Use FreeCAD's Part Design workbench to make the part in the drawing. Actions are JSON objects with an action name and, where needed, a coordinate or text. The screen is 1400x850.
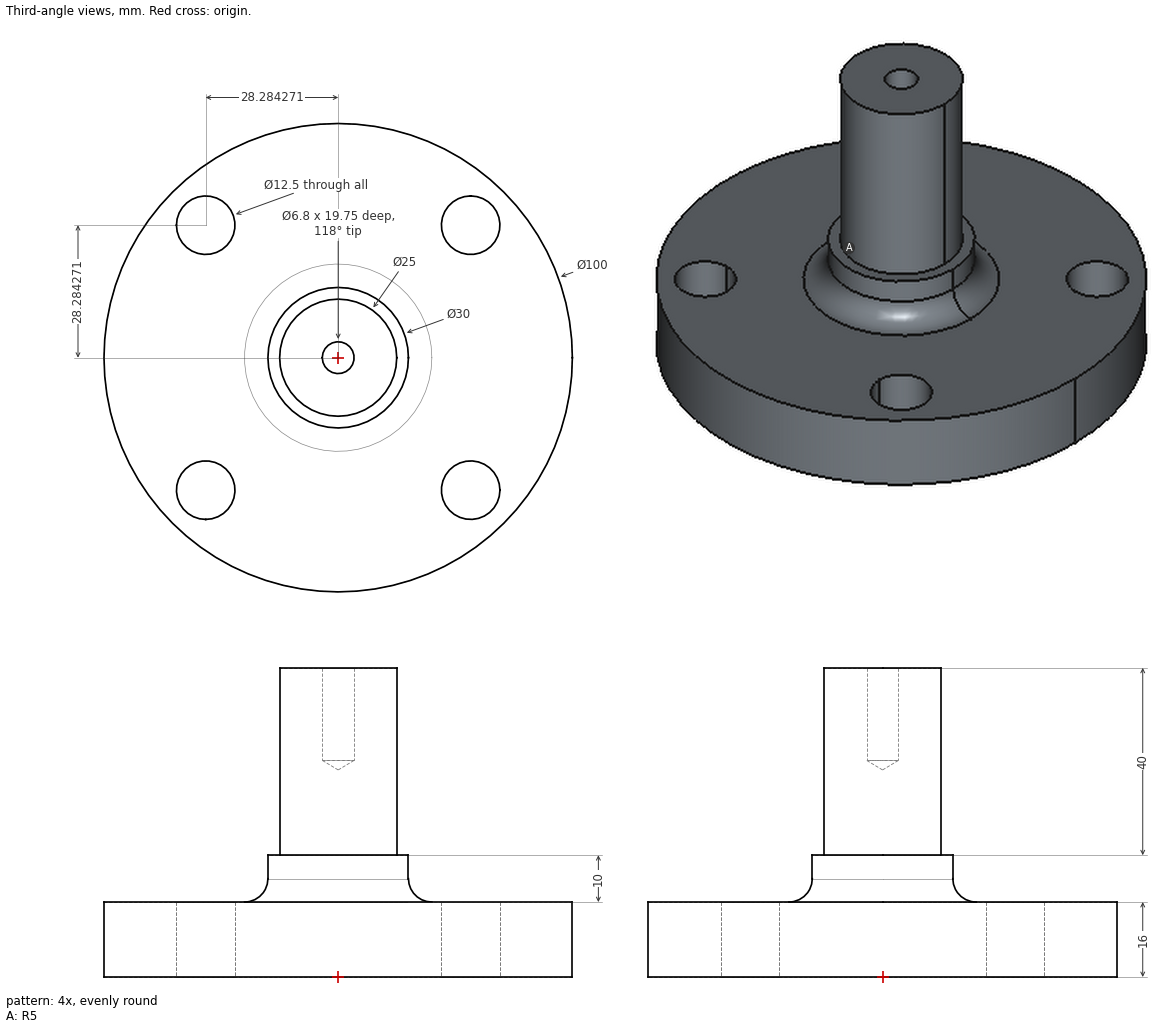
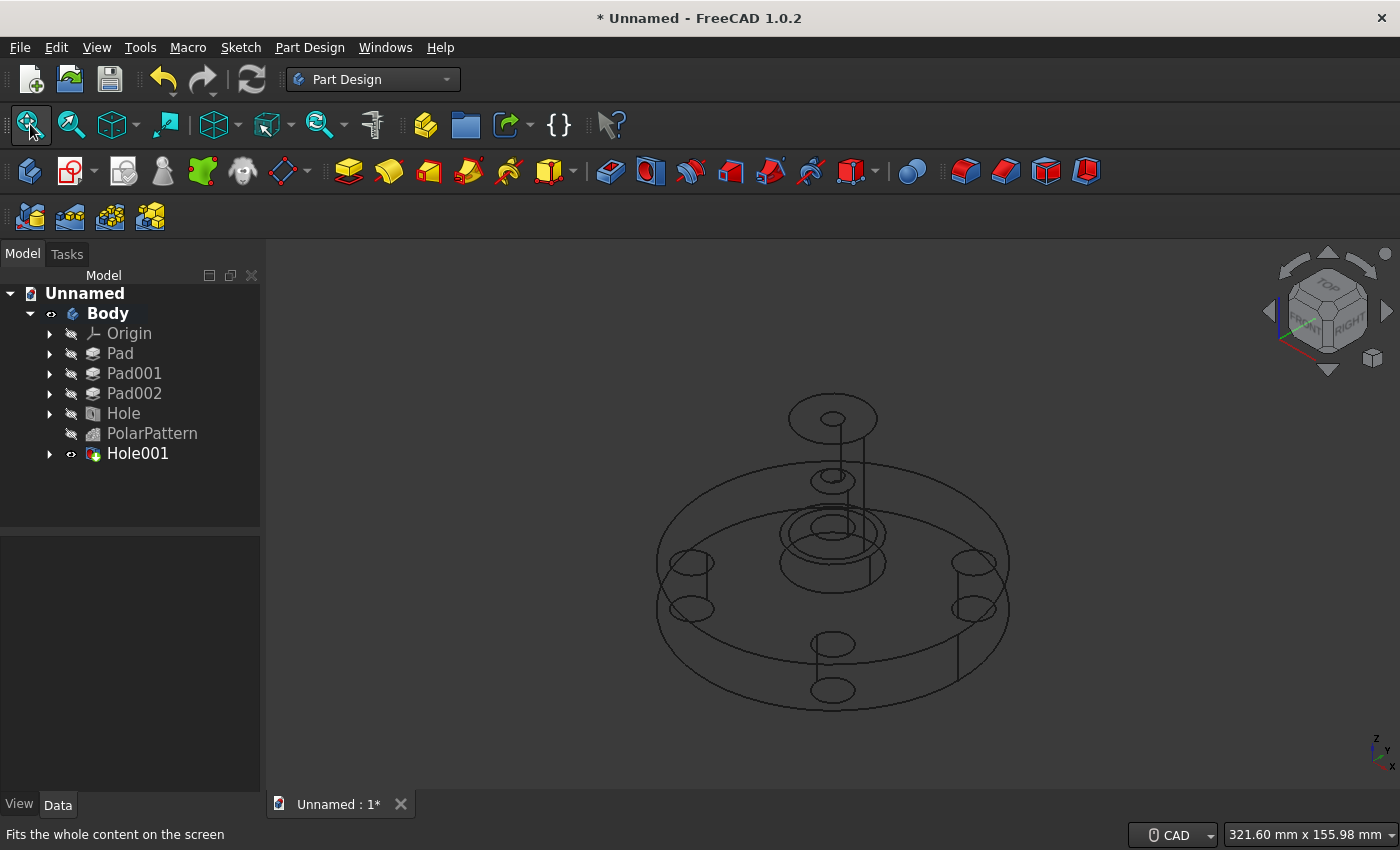
{"action": "left_click", "coordinate": [825, 532]}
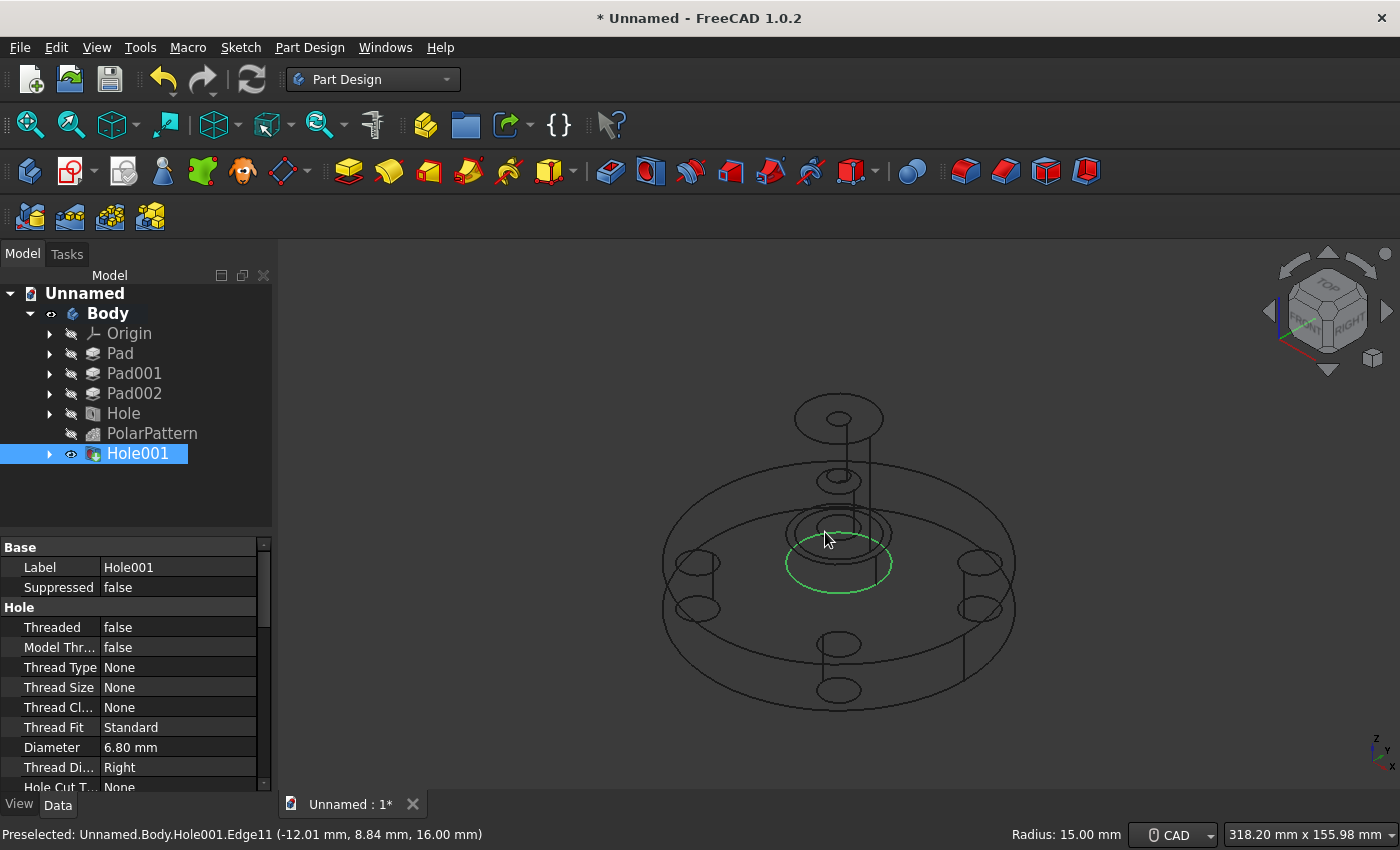
{"action": "key", "text": "v 1"}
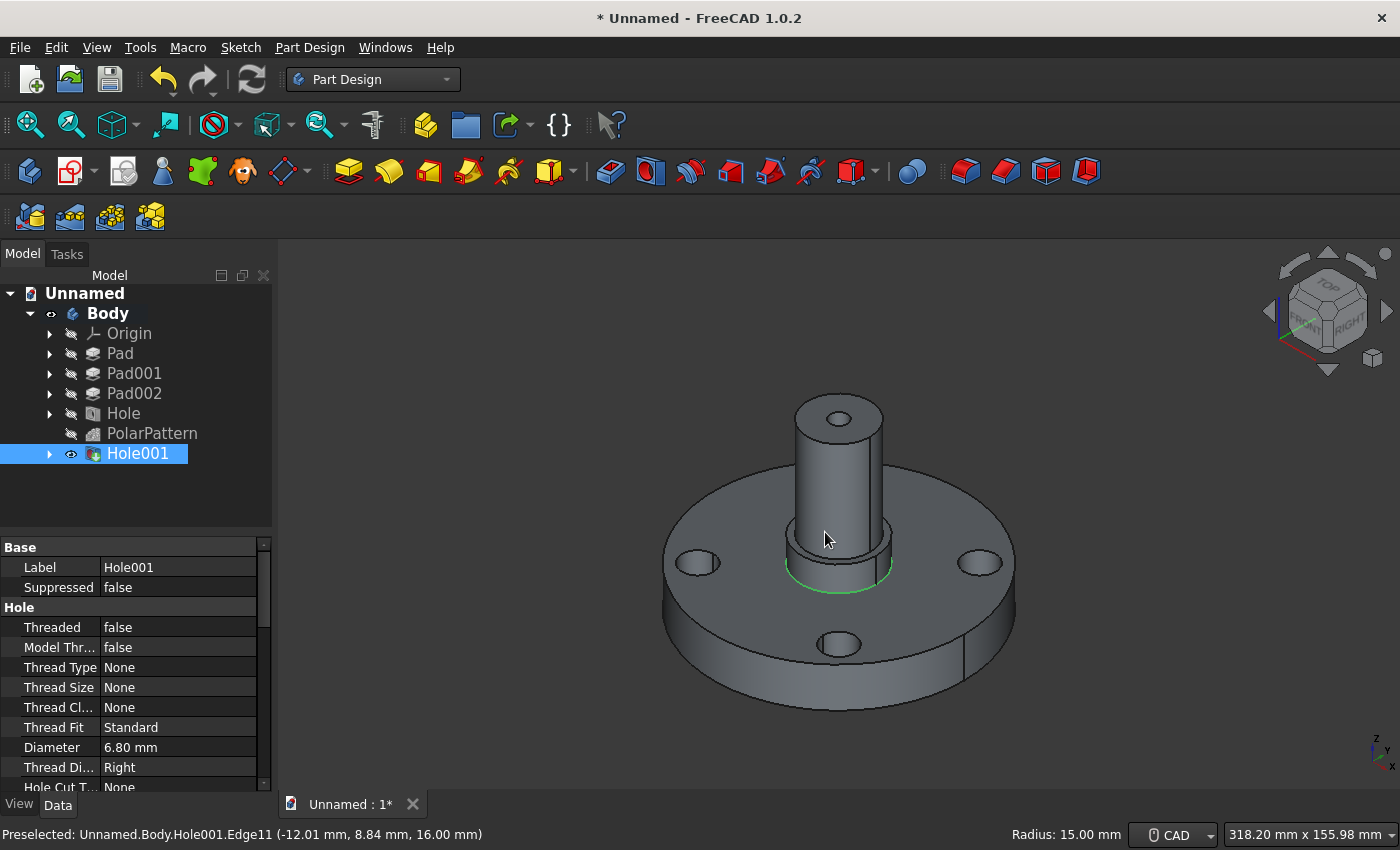
{"action": "left_click", "coordinate": [966, 172]}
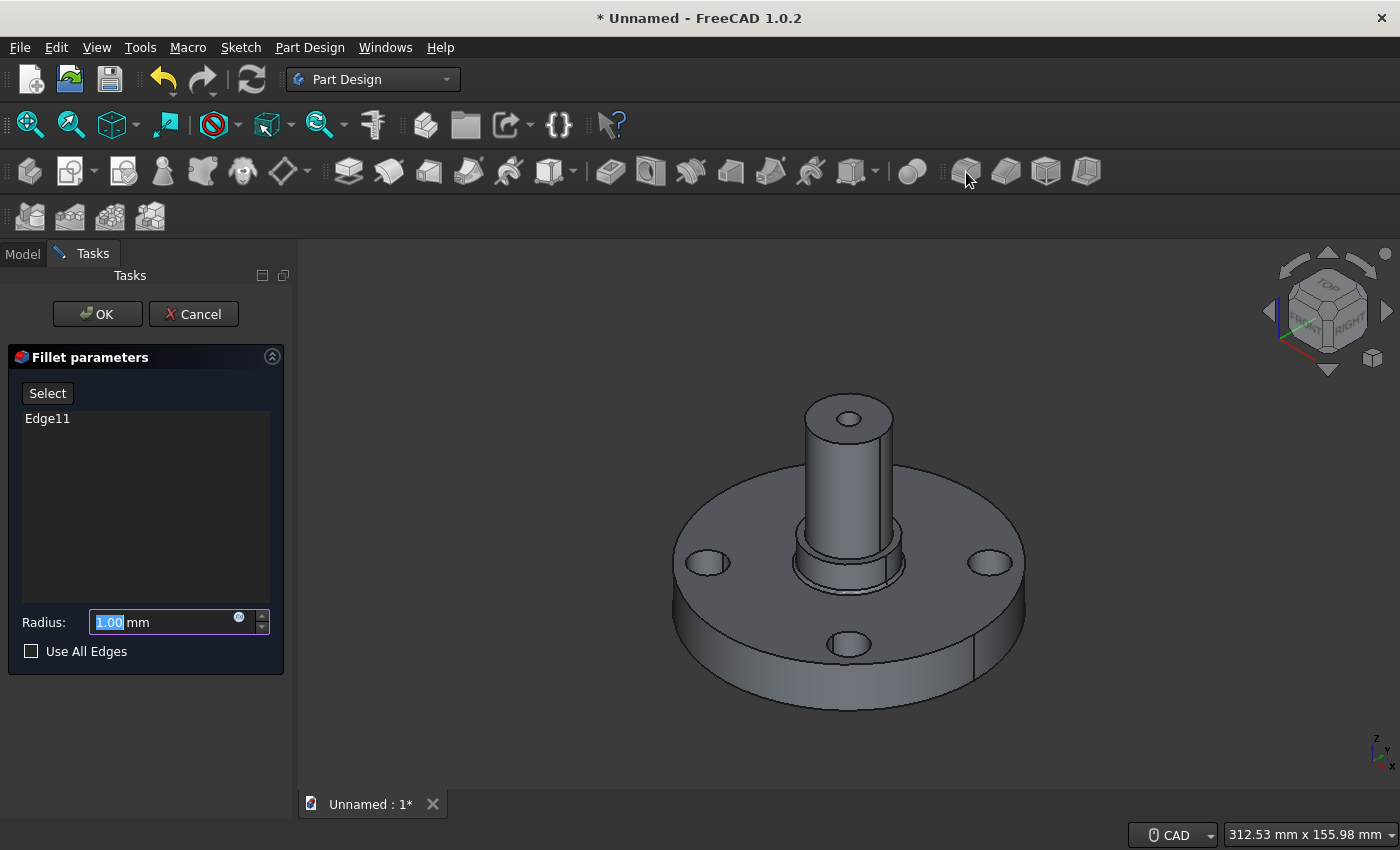
{"action": "type", "text": "5"}
{"action": "key", "text": "Tab"}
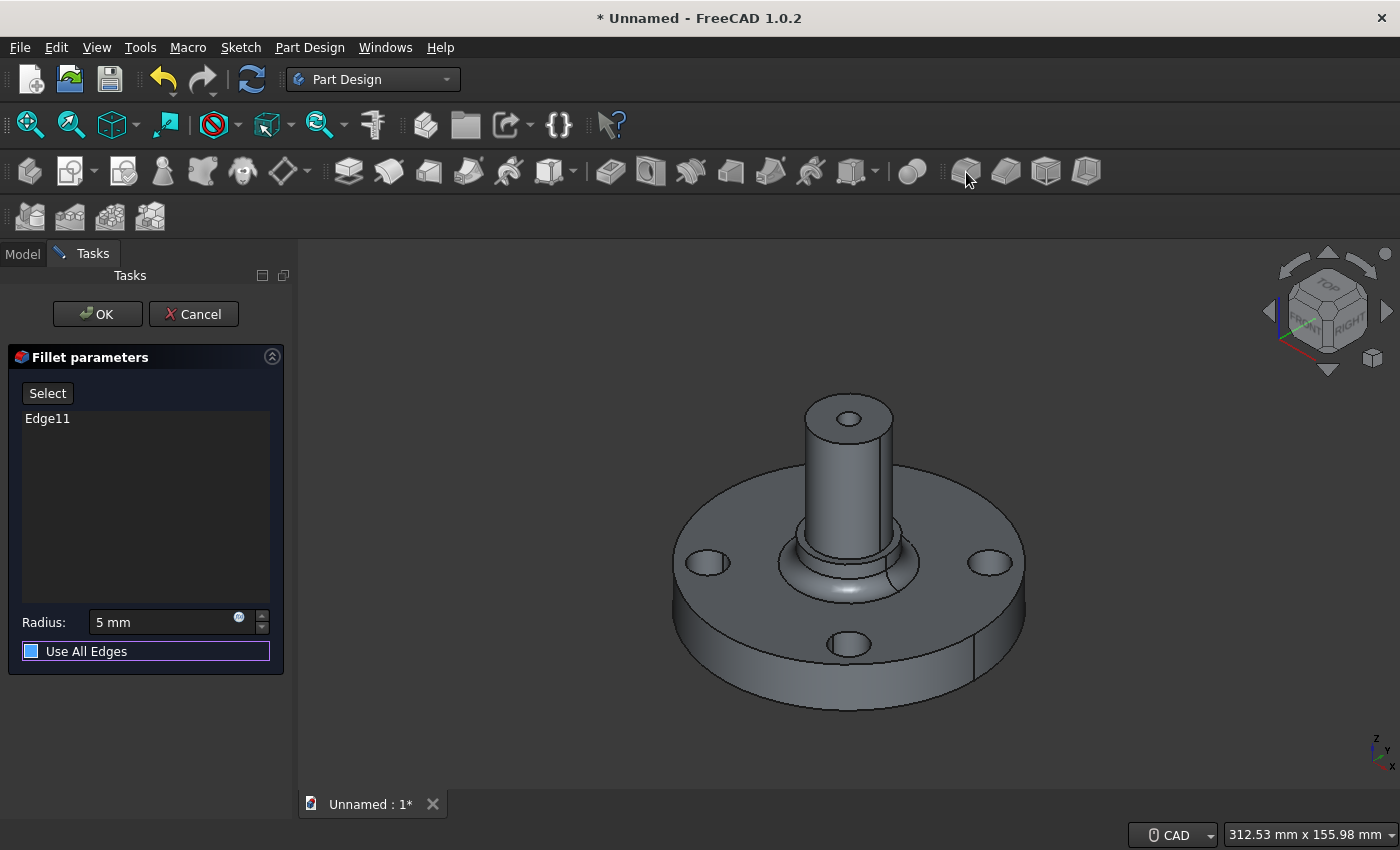
{"action": "left_click", "coordinate": [98, 314]}